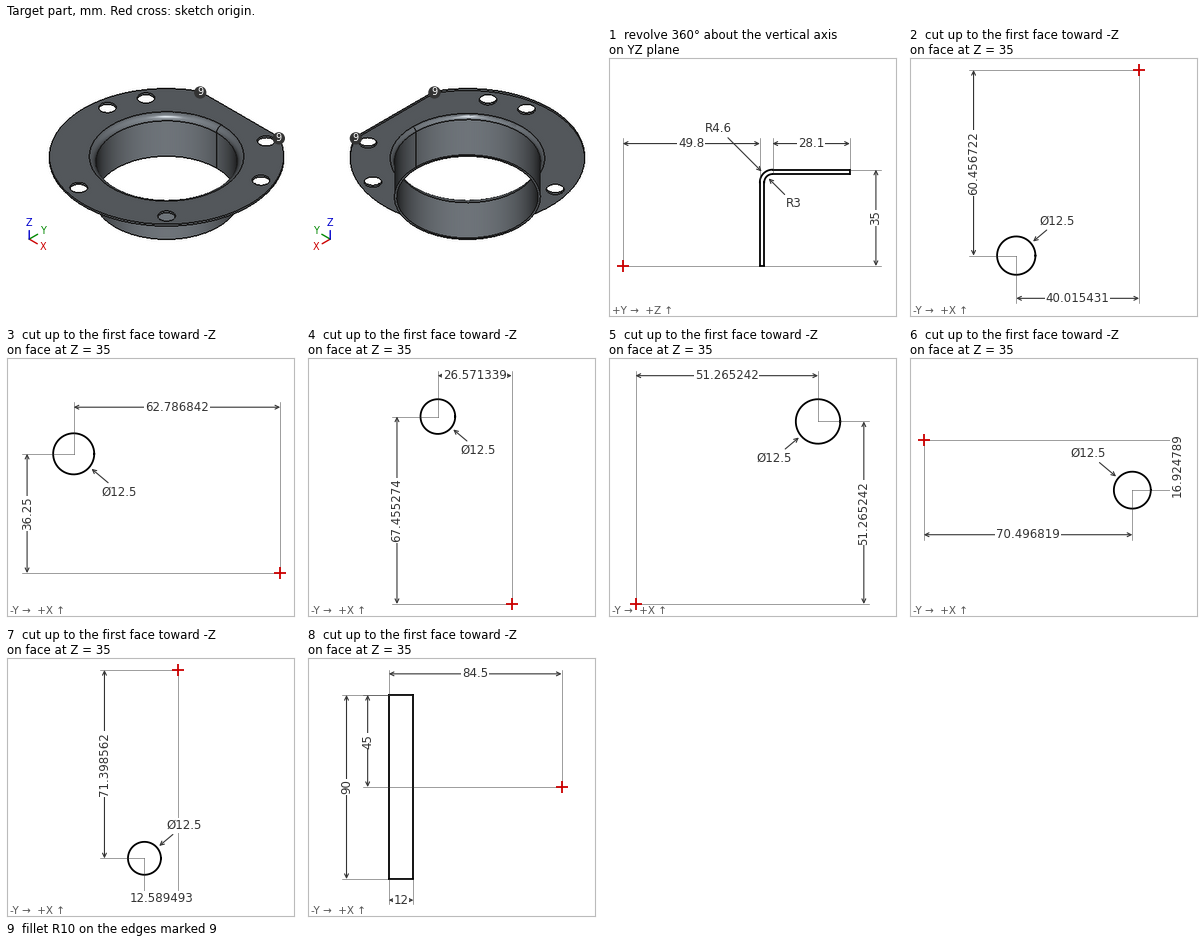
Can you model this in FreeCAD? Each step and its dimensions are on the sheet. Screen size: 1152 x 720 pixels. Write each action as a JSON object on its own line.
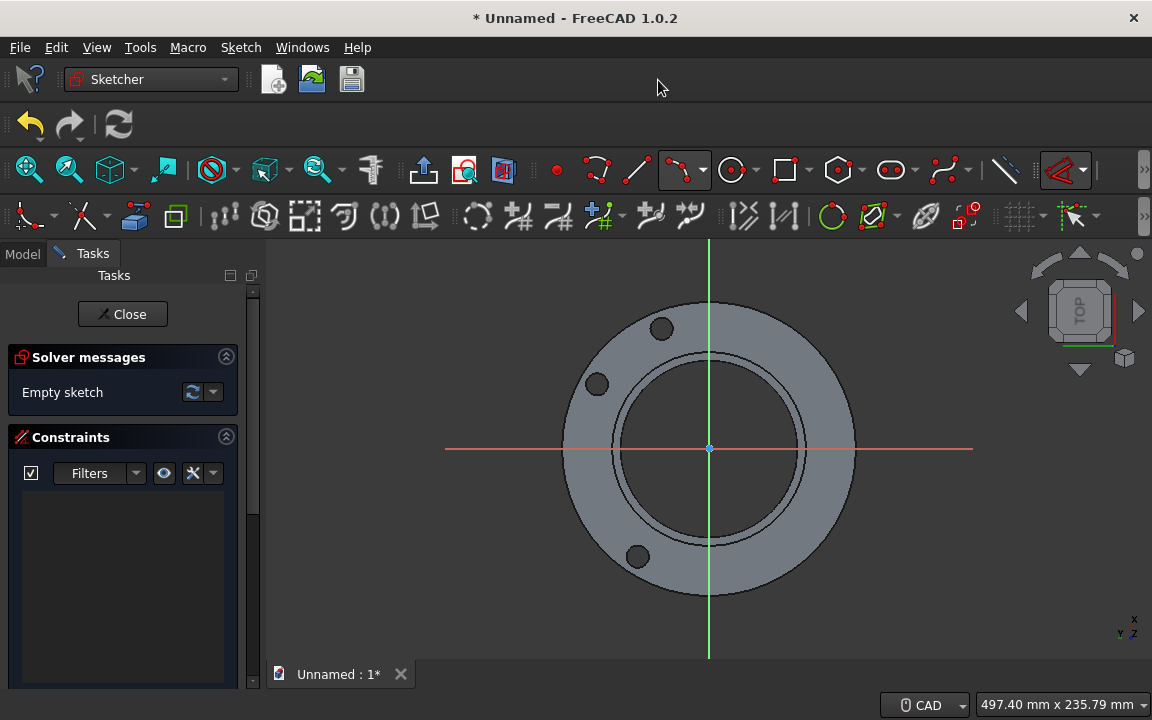
{"action": "scroll", "coordinate": [816, 349], "scroll_direction": "up", "scroll_amount": 12}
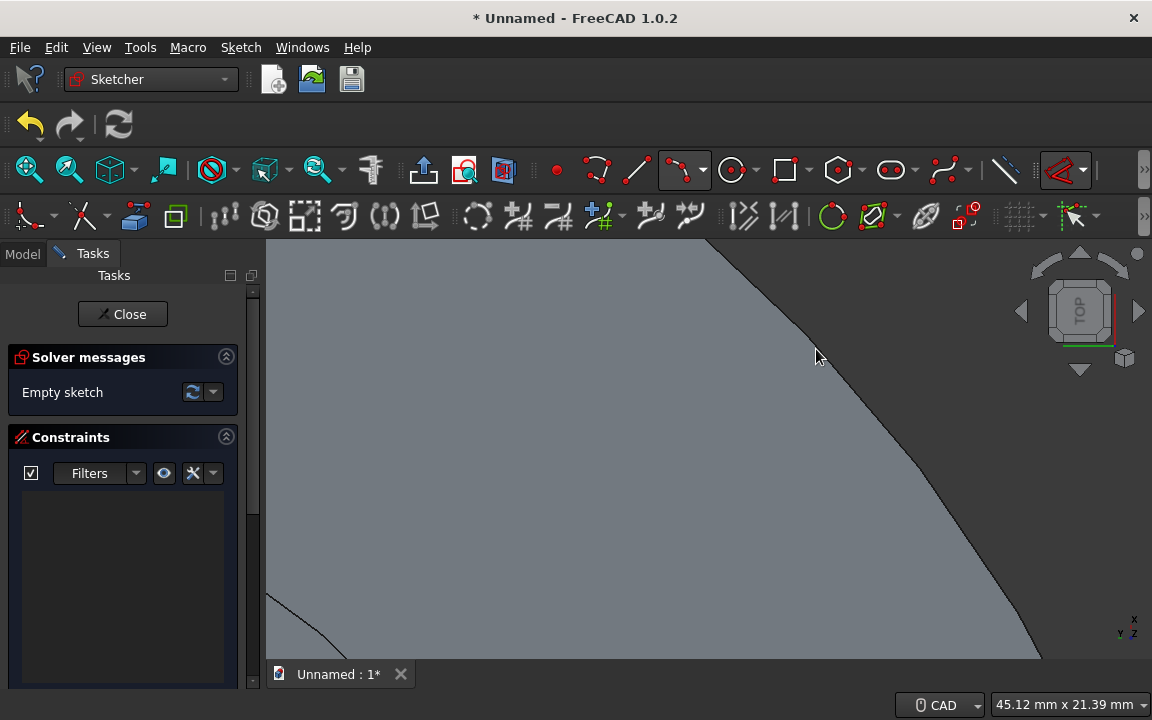
{"action": "key", "text": "g c"}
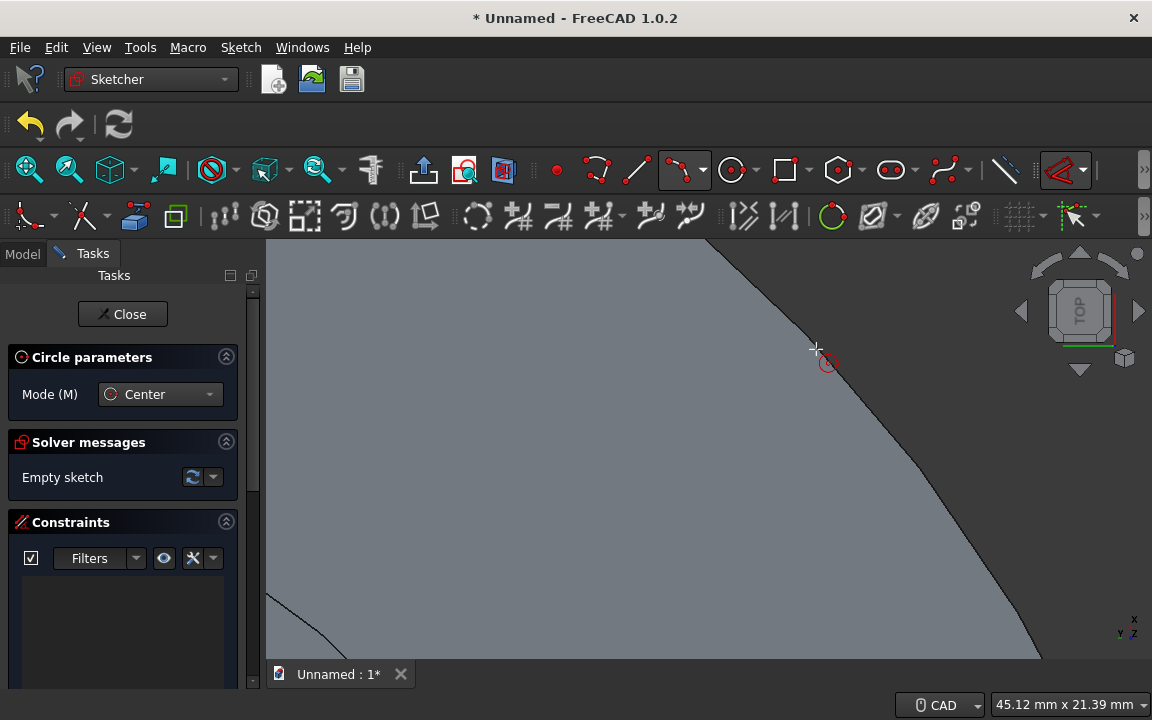
{"action": "left_click", "coordinate": [637, 442]}
{"action": "mouse_move", "coordinate": [724, 355]}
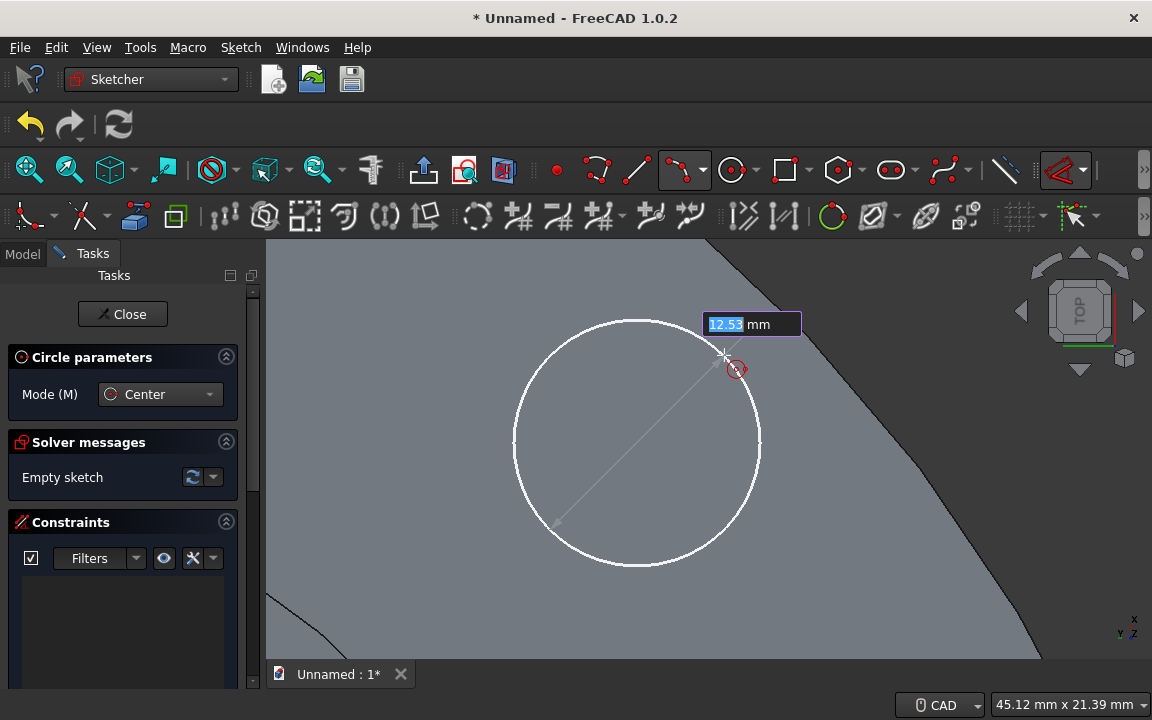
{"action": "type", "text": "12.5"}
{"action": "key", "text": "Return"}
{"action": "key", "text": "Escape"}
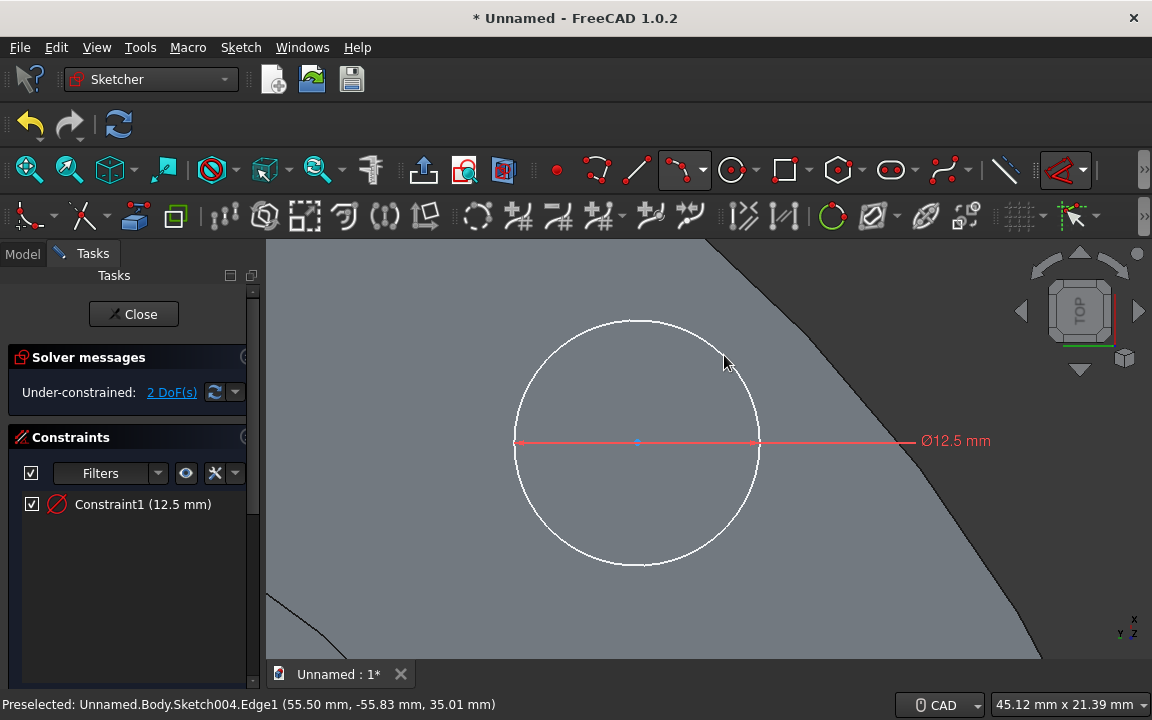
{"action": "left_click", "coordinate": [637, 443]}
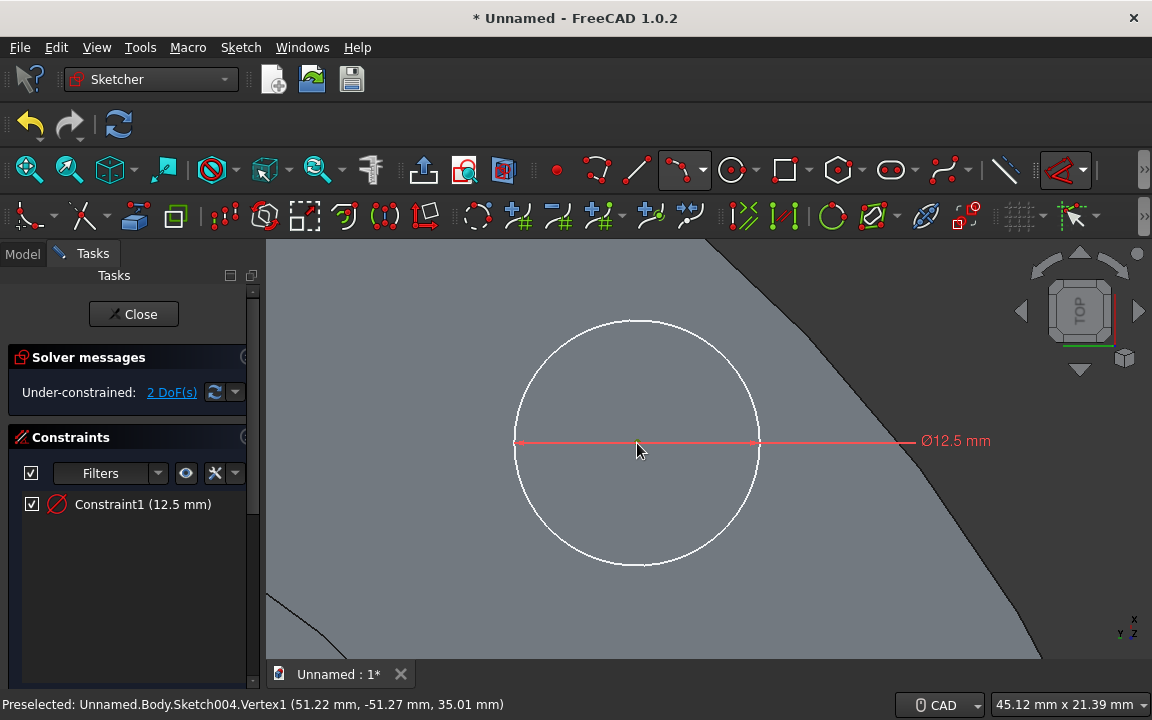
{"action": "key", "text": "l"}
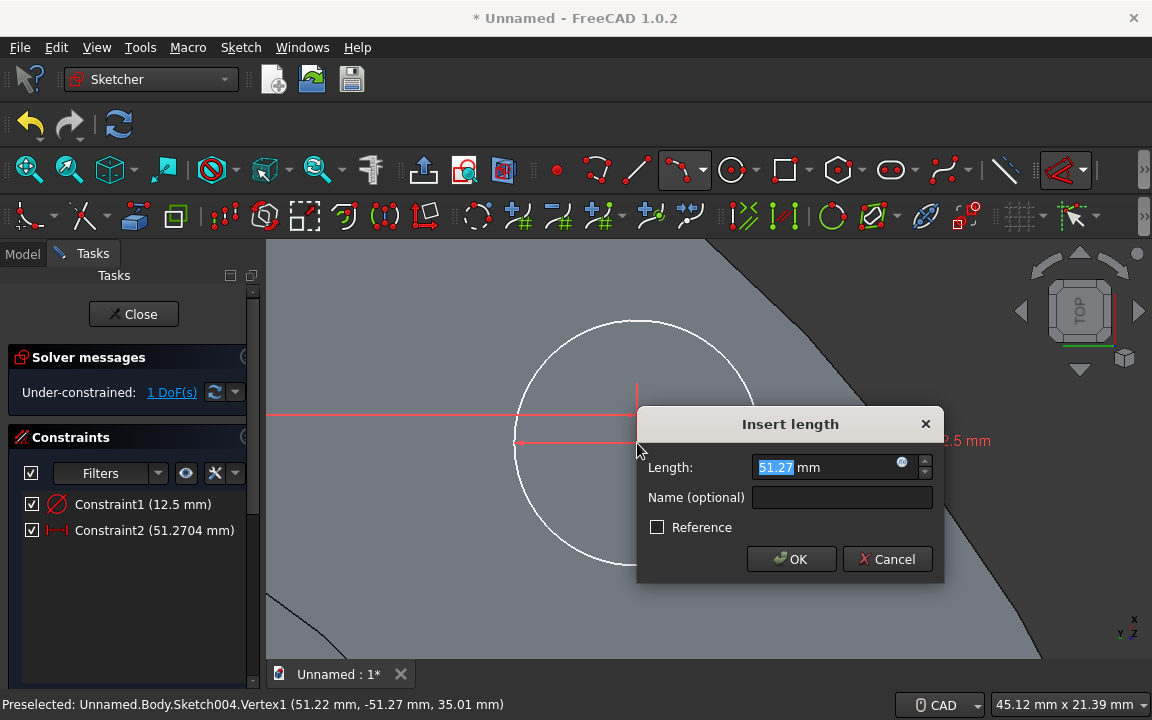
{"action": "type", "text": "51.265242"}
{"action": "key", "text": "Return"}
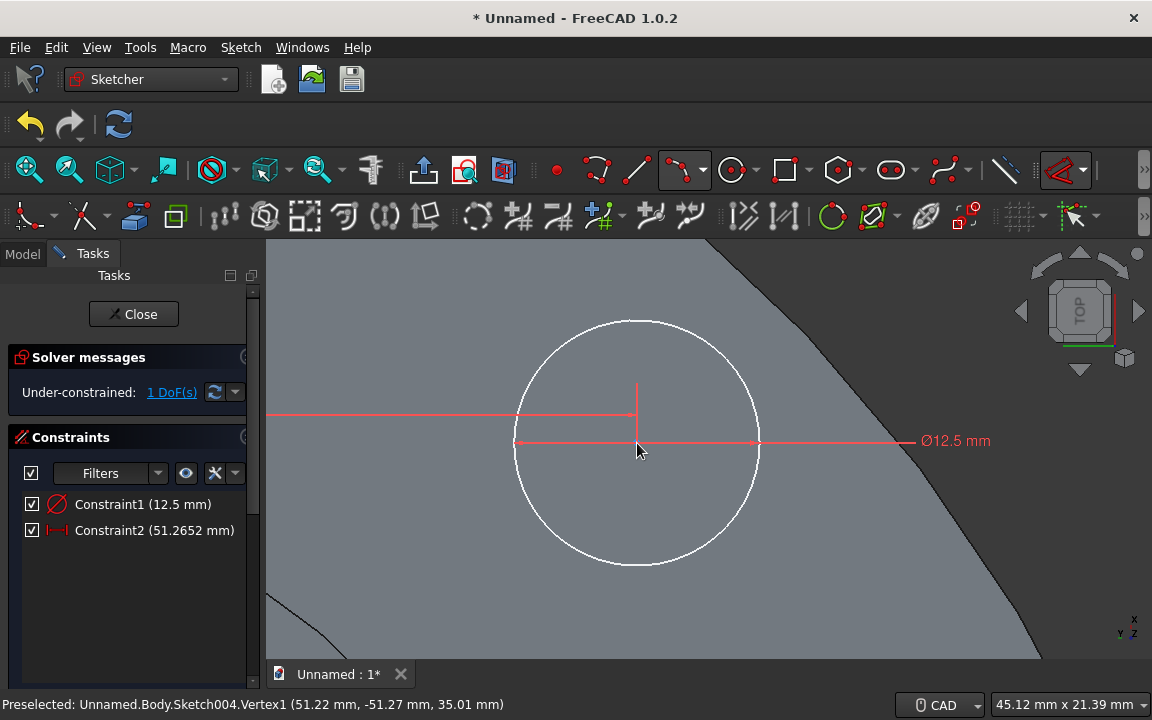
{"action": "left_click", "coordinate": [637, 443]}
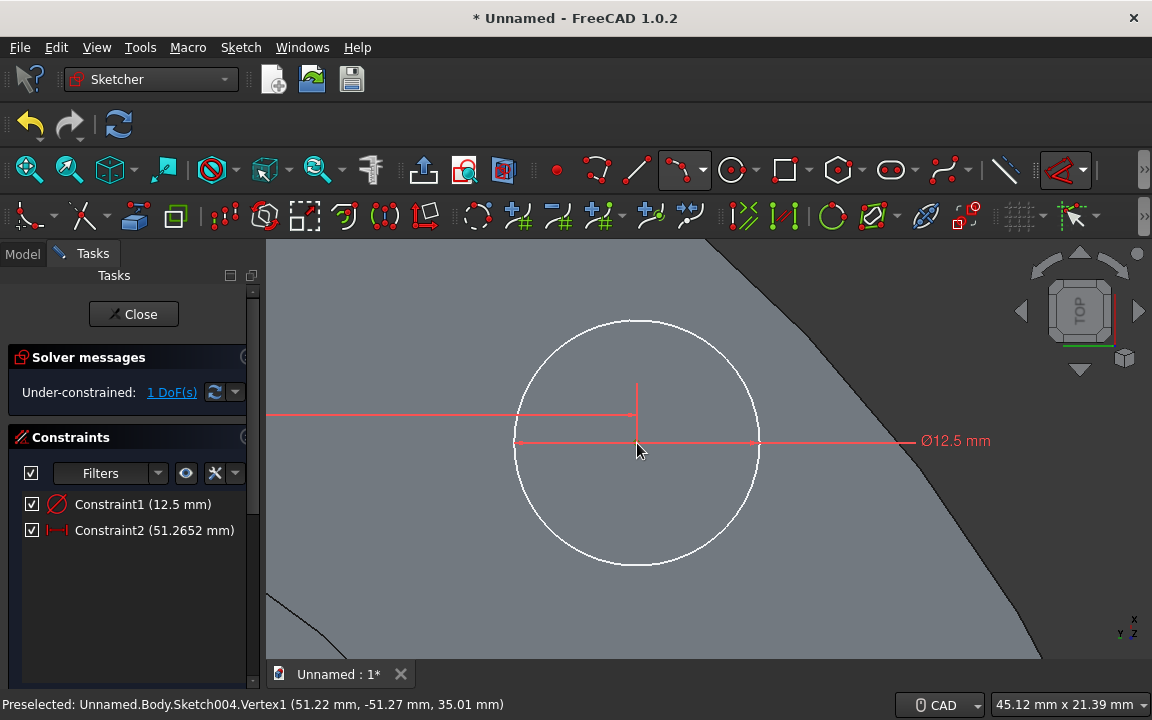
{"action": "key", "text": "i"}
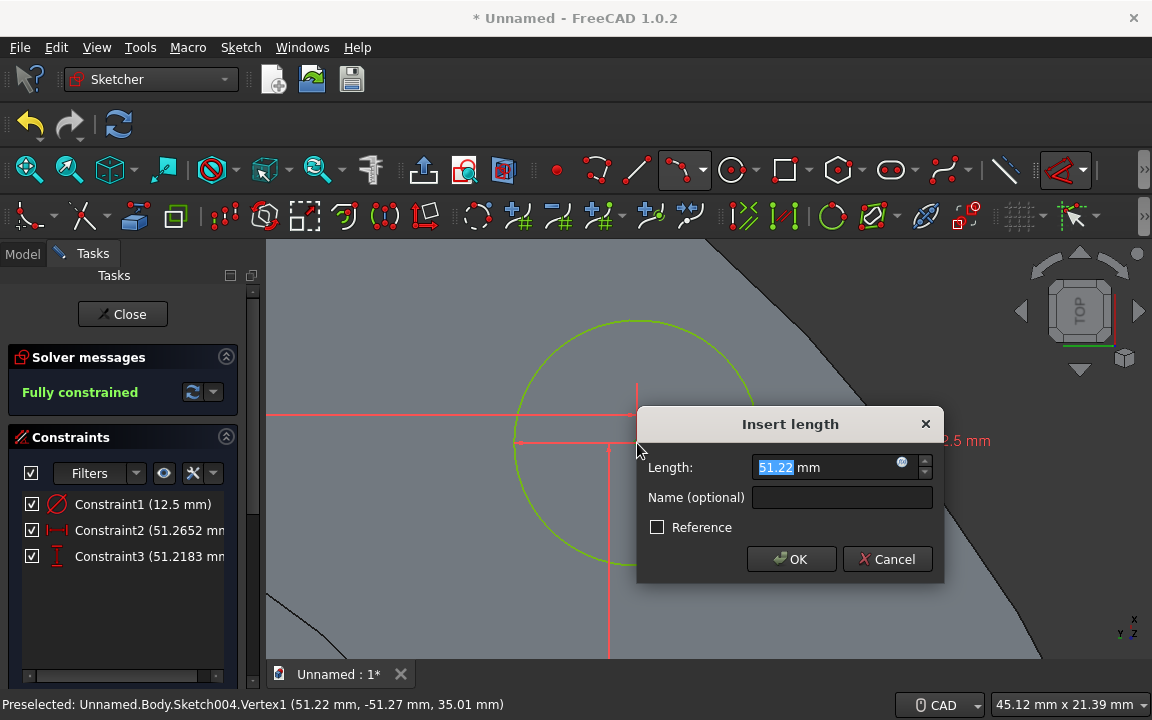
{"action": "type", "text": "51.265242"}
{"action": "key", "text": "Return"}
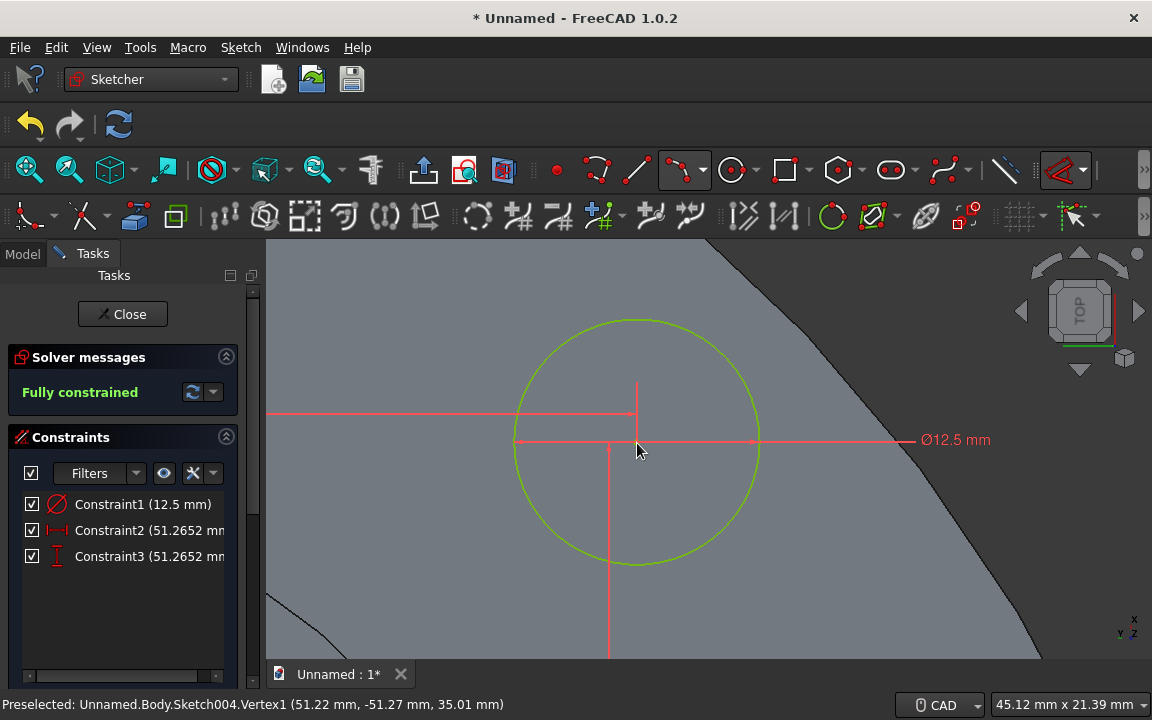
{"action": "left_click", "coordinate": [123, 314]}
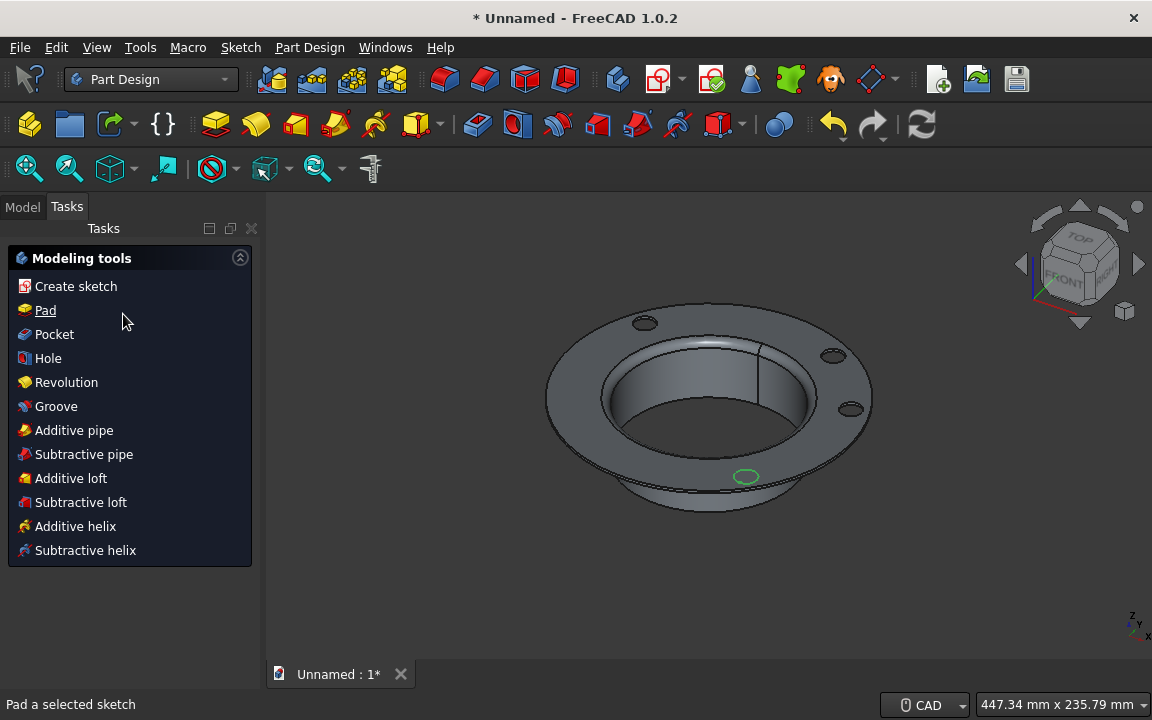
{"action": "left_click", "coordinate": [478, 124]}